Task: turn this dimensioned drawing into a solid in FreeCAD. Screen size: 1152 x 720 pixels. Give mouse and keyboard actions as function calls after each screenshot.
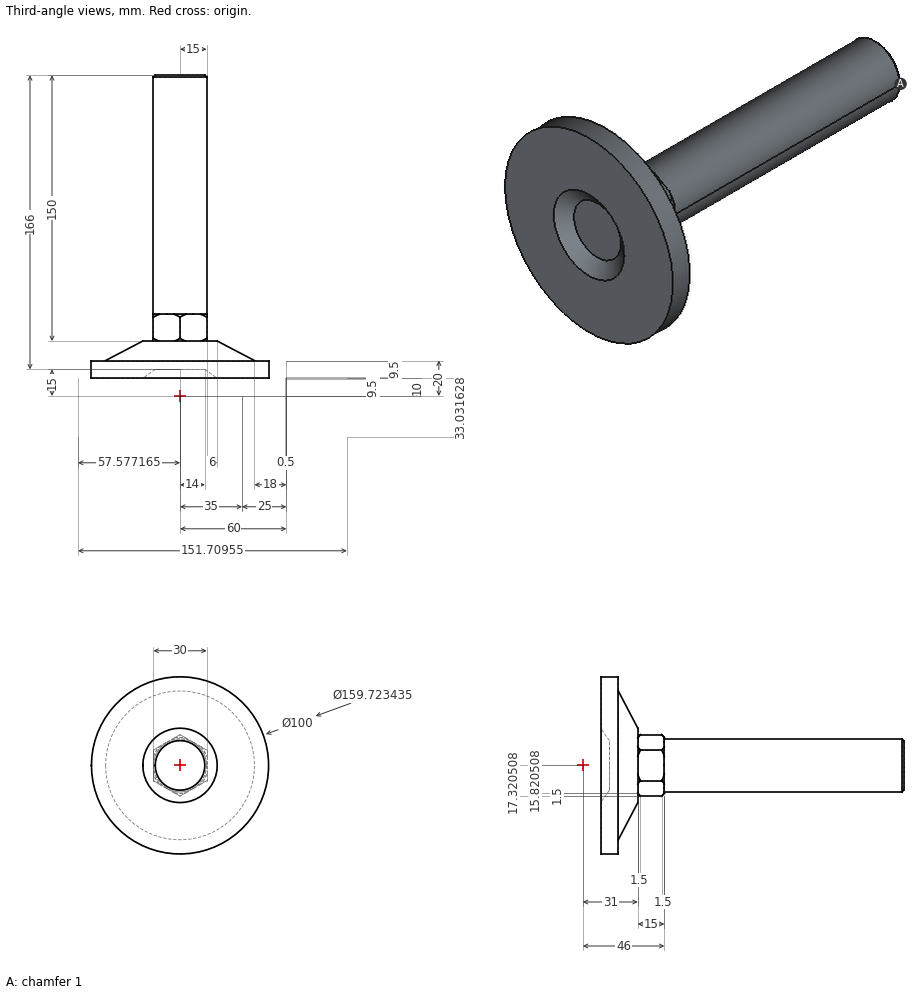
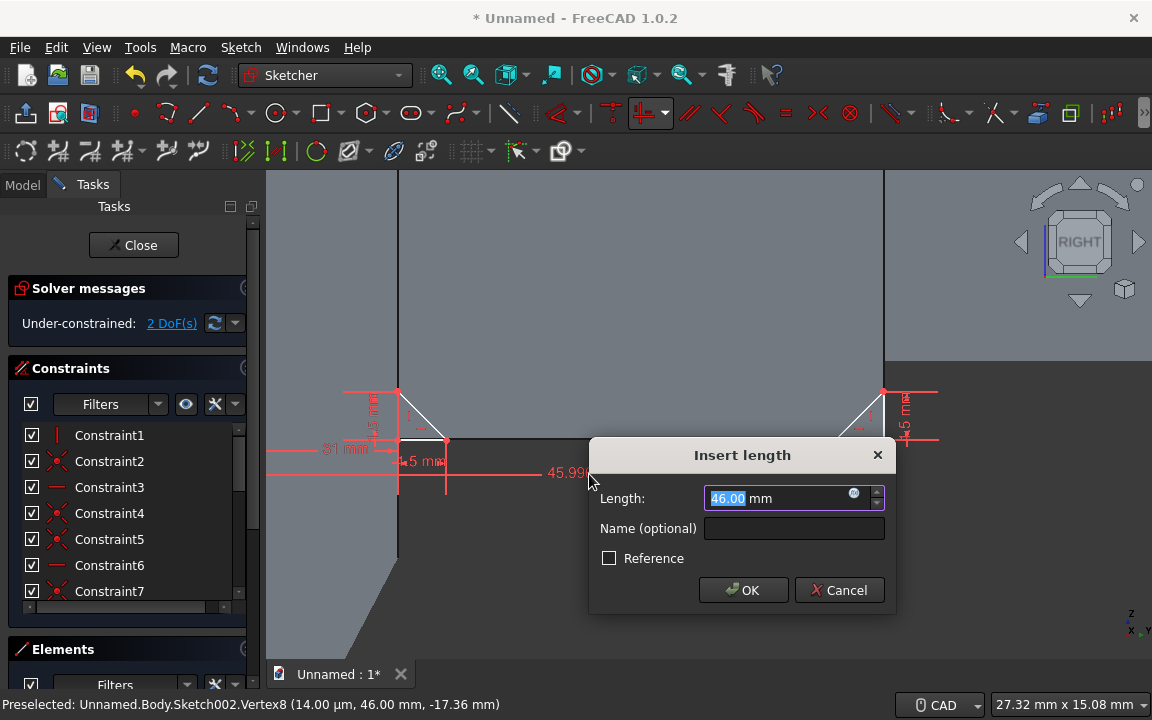
text(46)
key(Return)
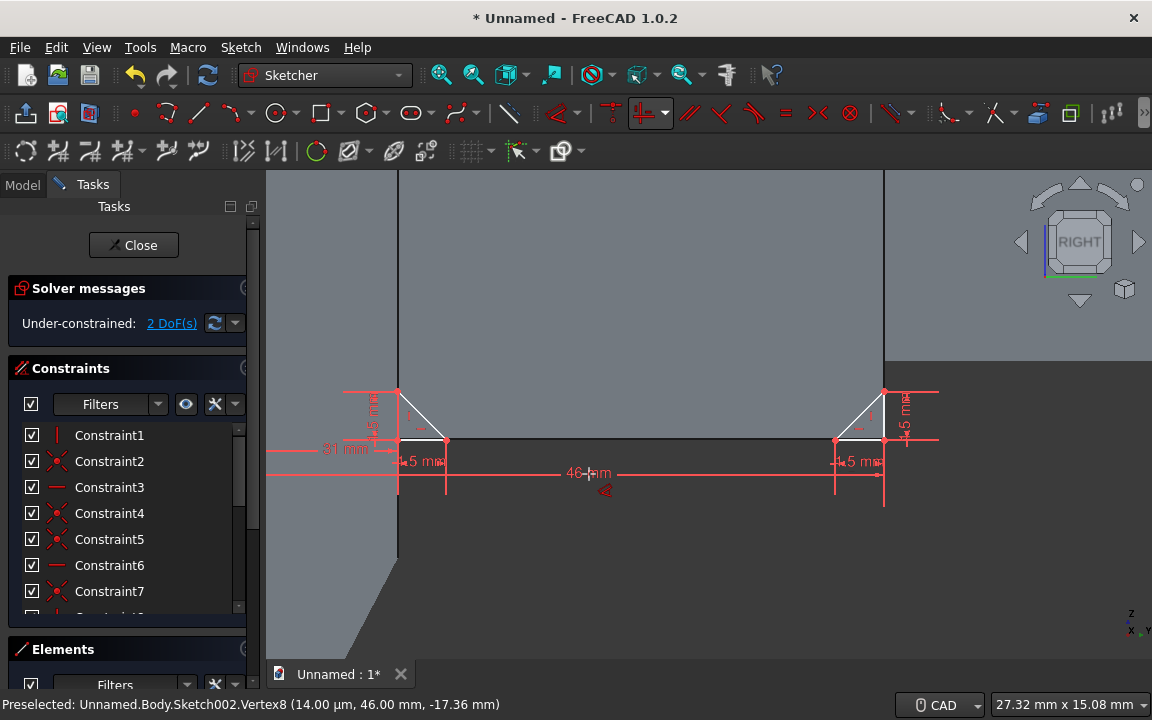
click(398, 392)
click(432, 295)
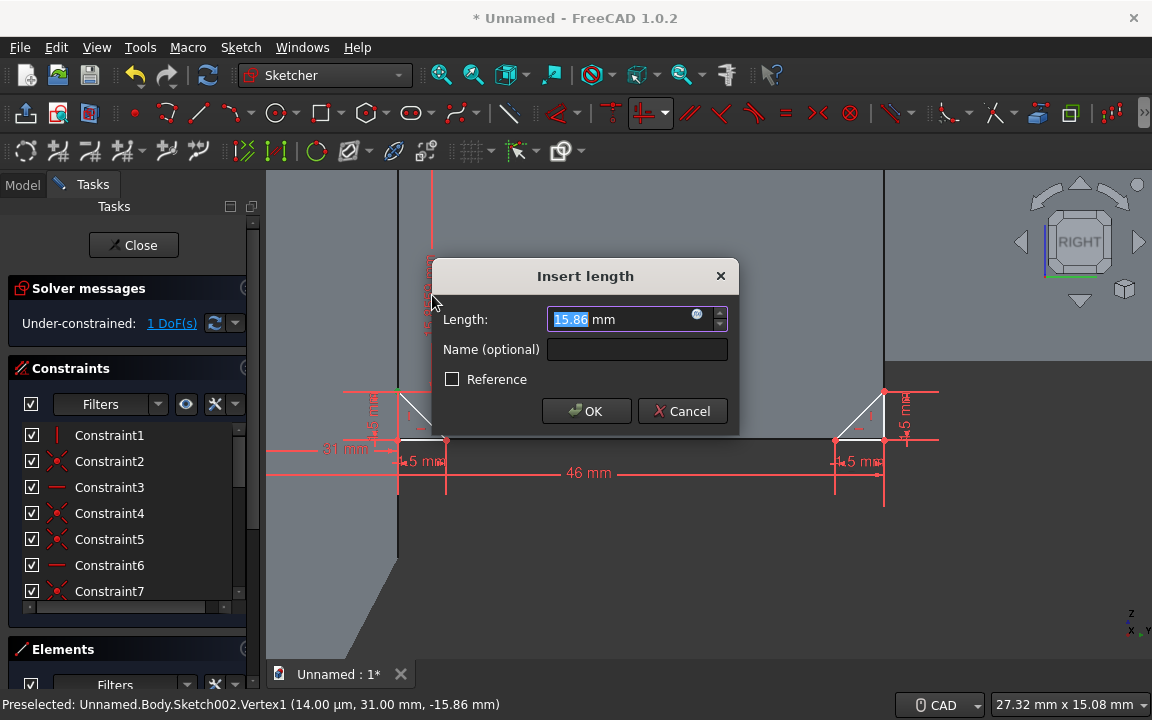
text(15.820508)
key(Return)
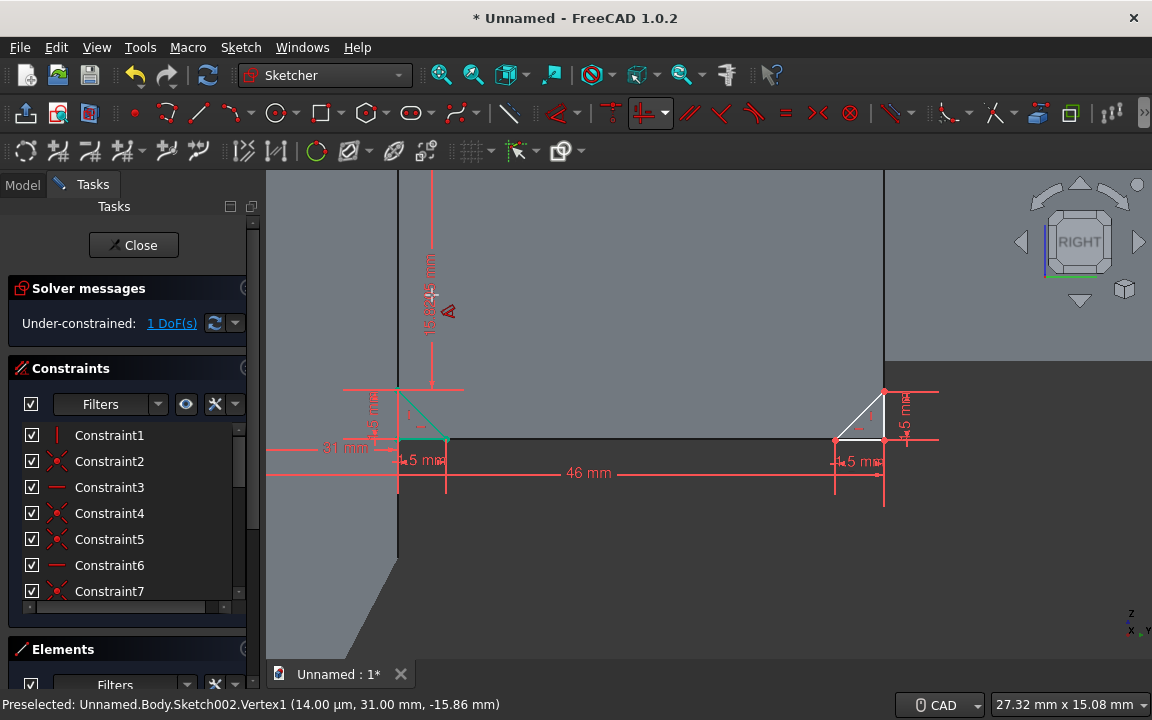
click(835, 440)
click(869, 319)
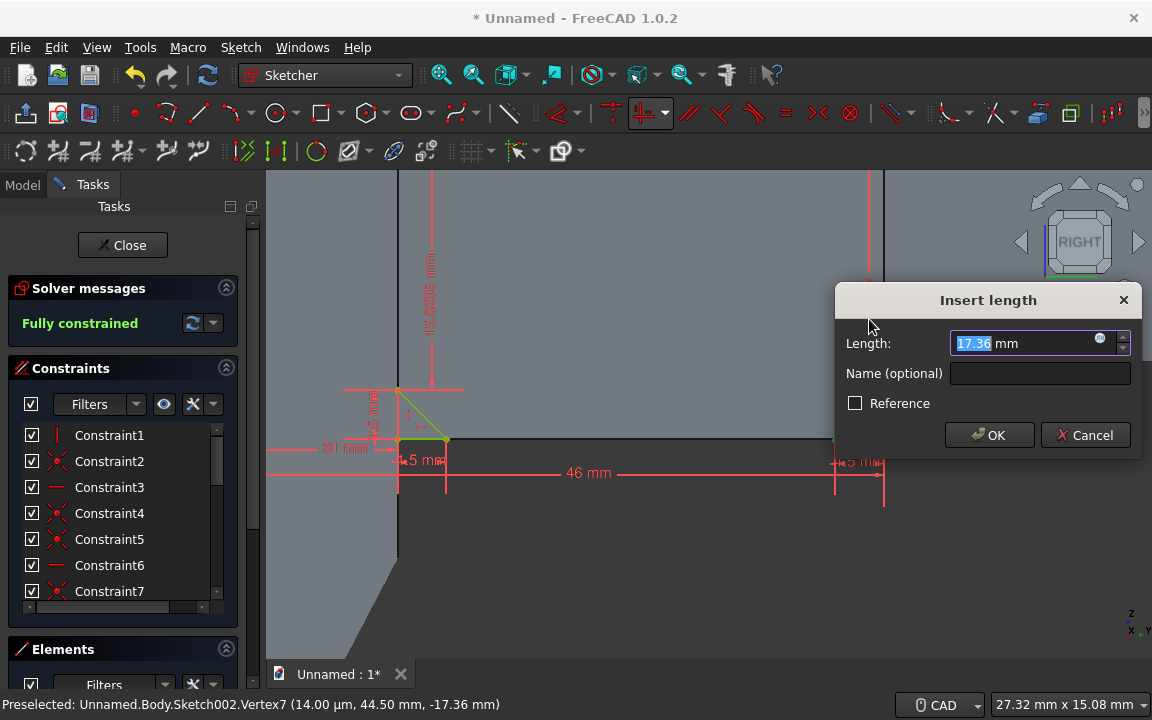
text(17.320508)
key(Return)
key(Escape)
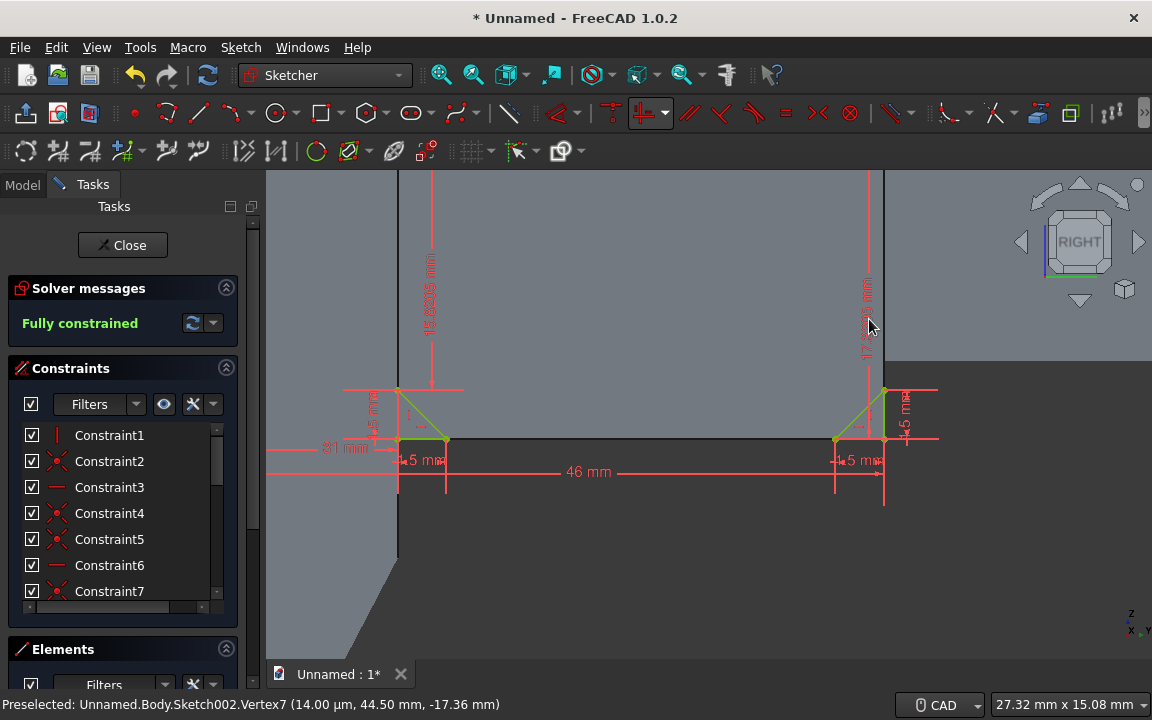
click(123, 245)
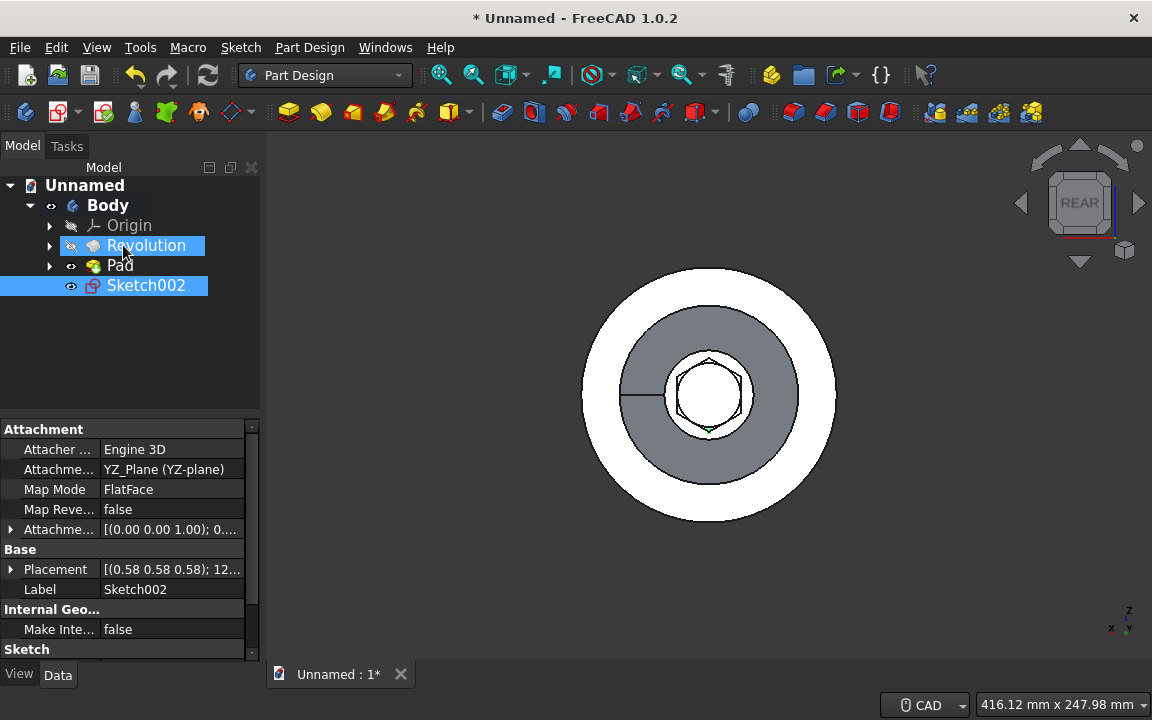
click(568, 112)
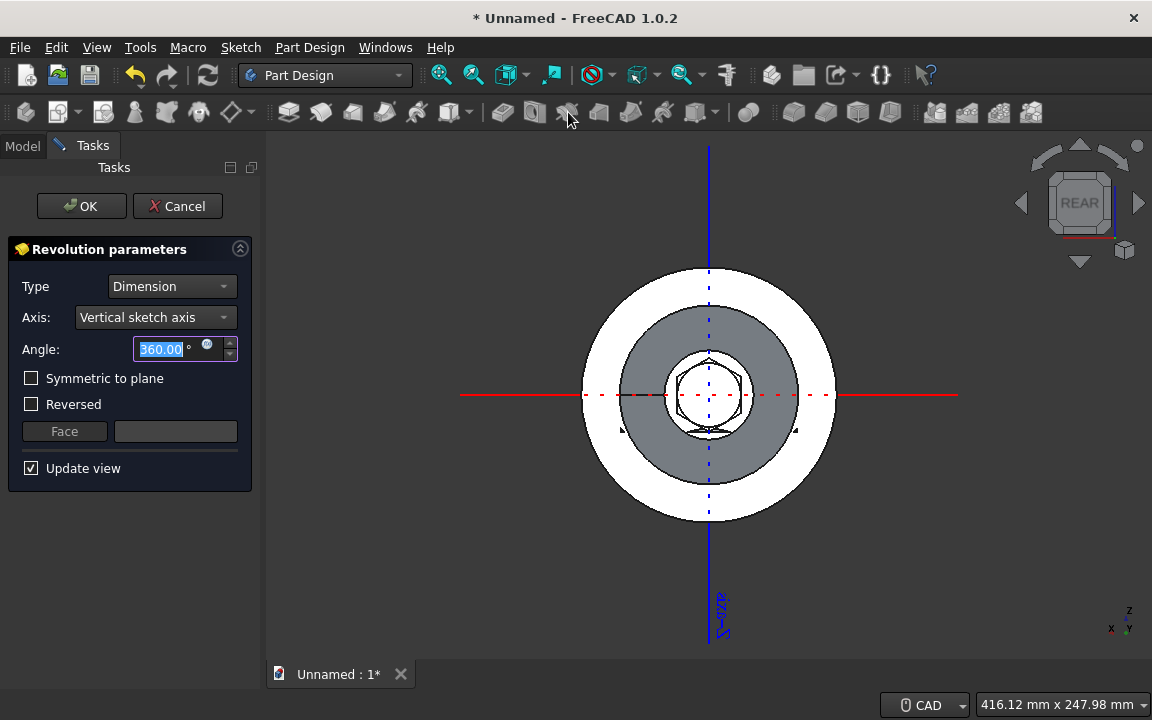
click(156, 318)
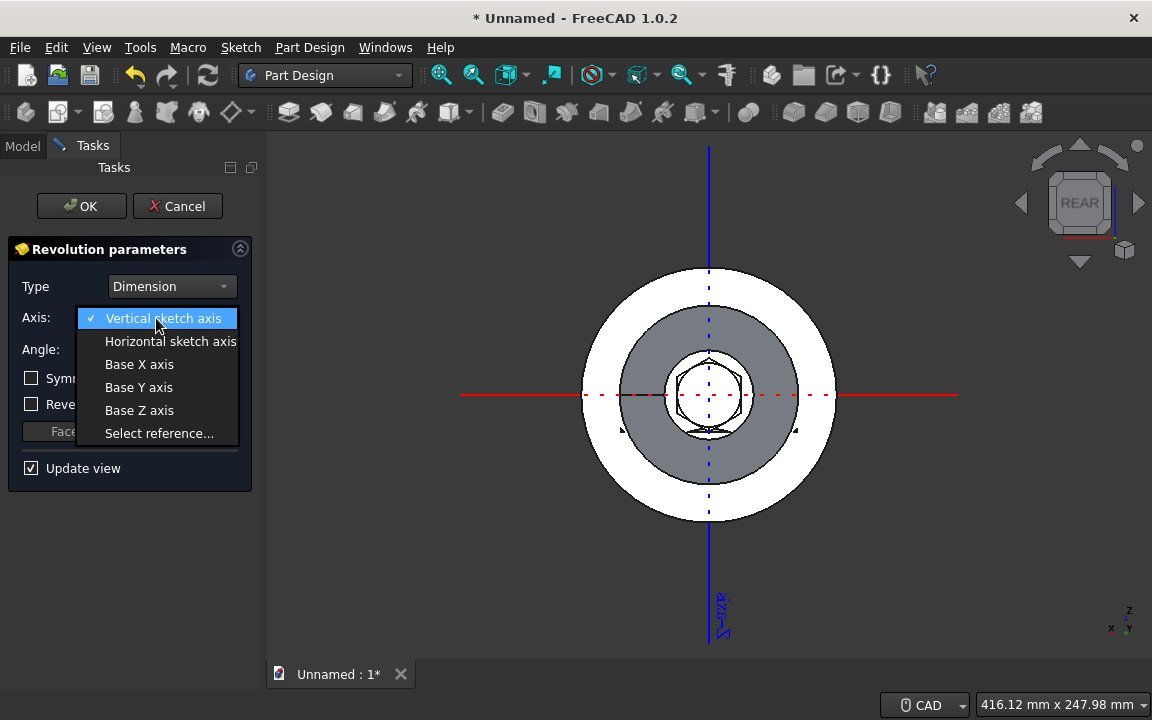
click(156, 342)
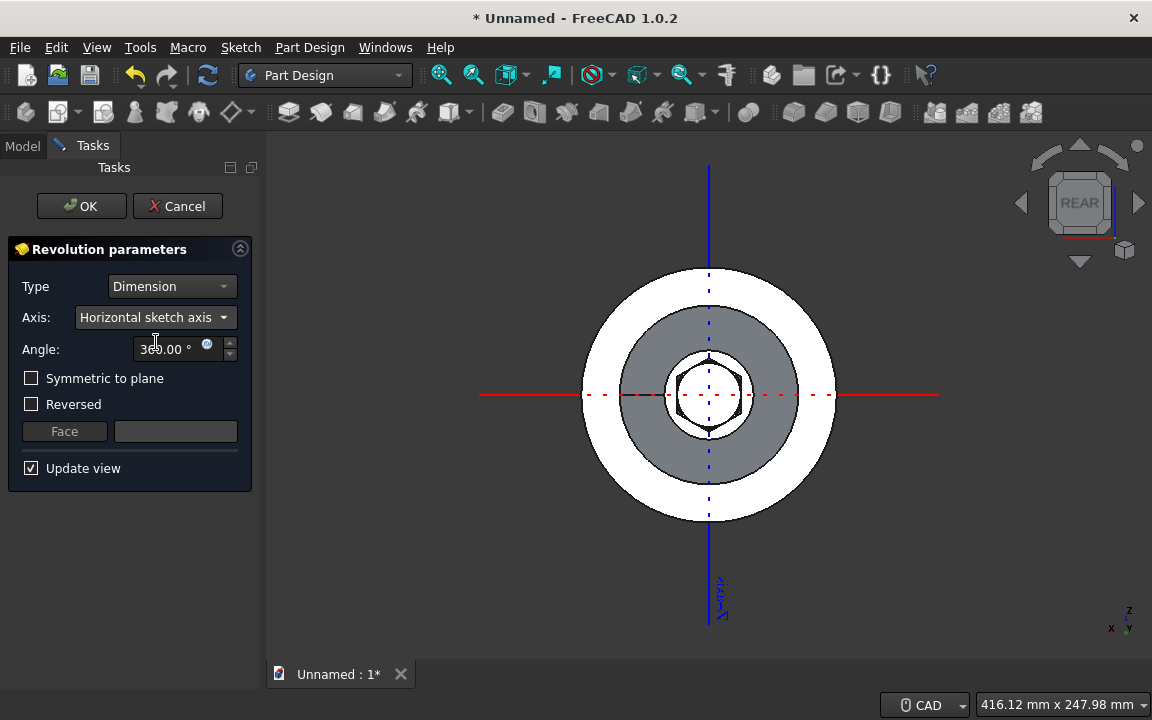
click(82, 206)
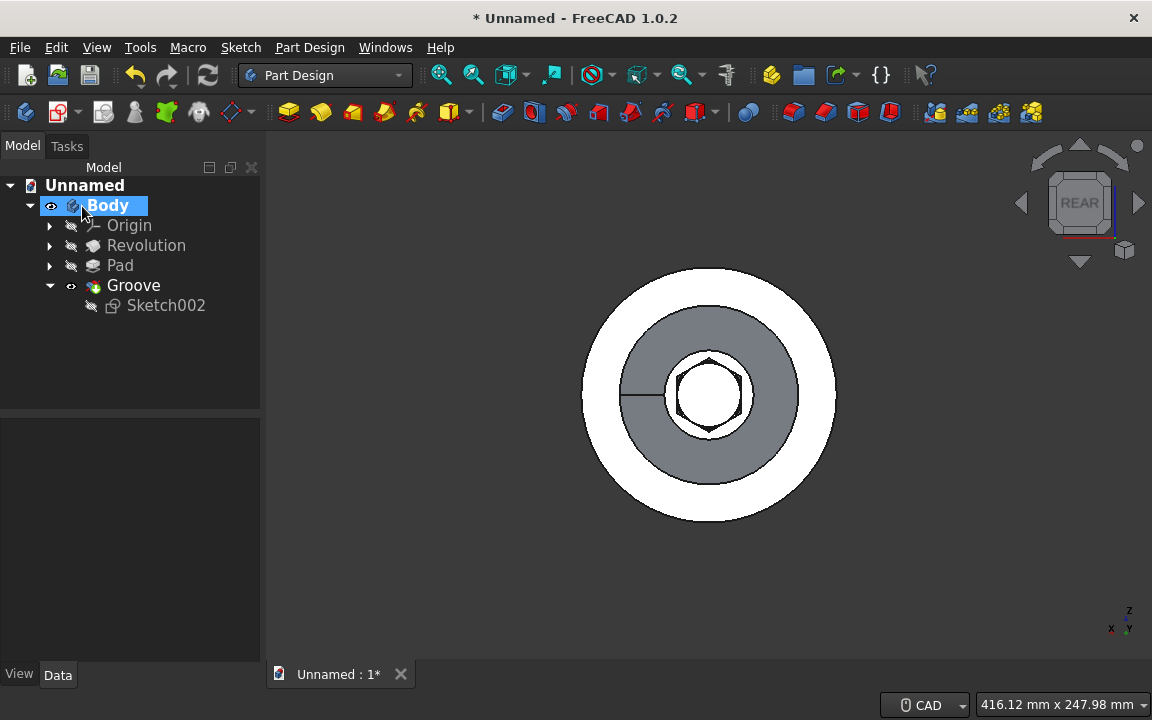
click(741, 394)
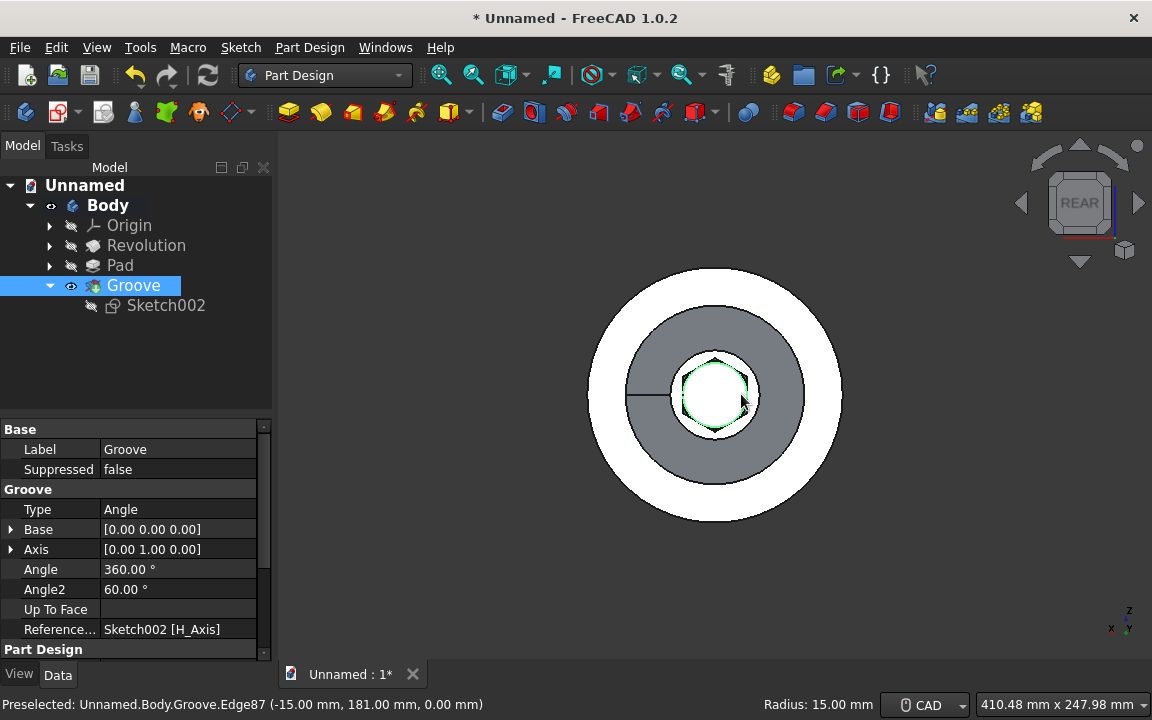
click(826, 112)